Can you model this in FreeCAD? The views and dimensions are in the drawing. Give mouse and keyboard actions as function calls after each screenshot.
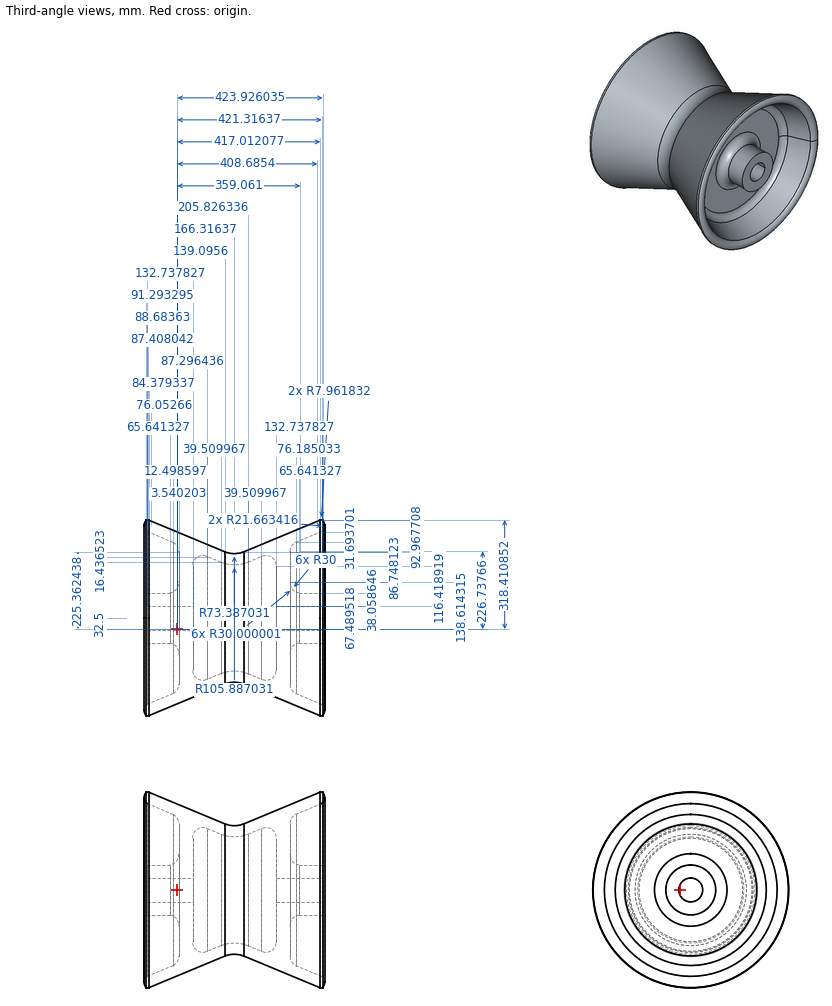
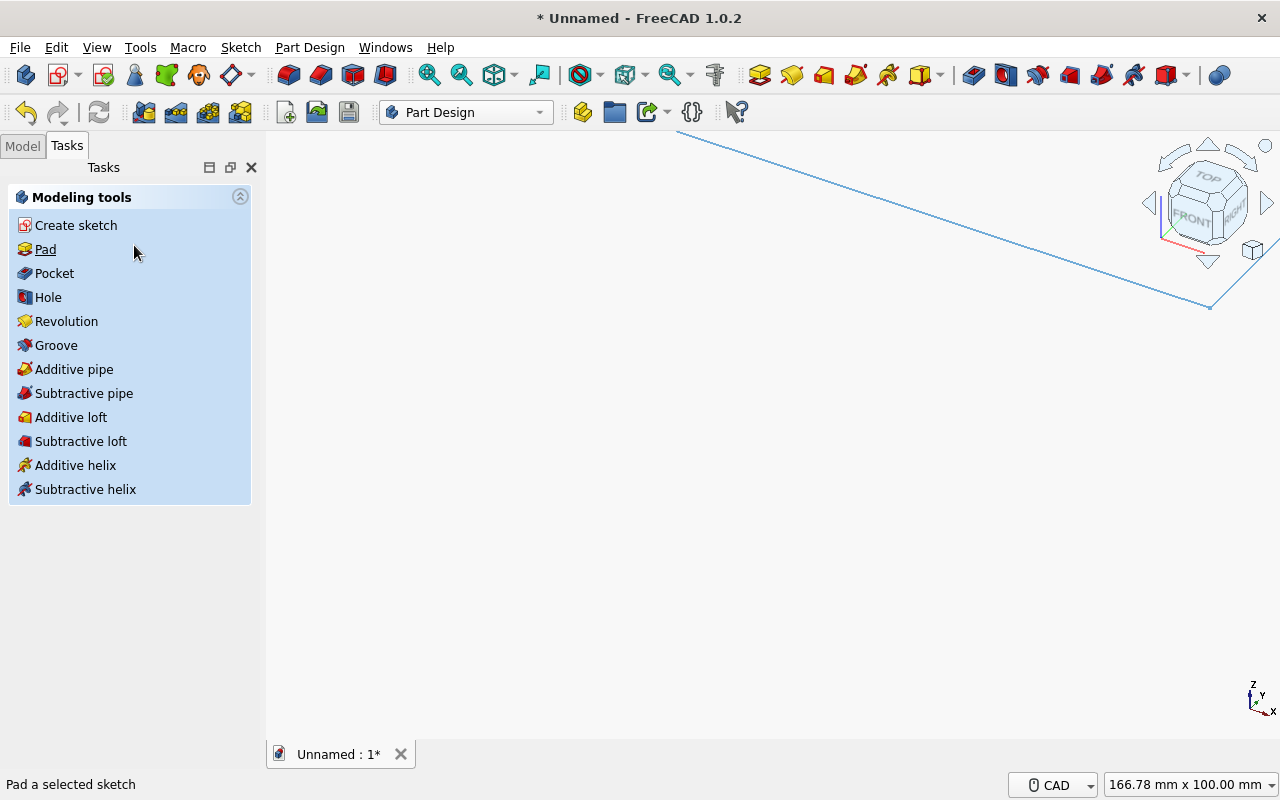
click(792, 76)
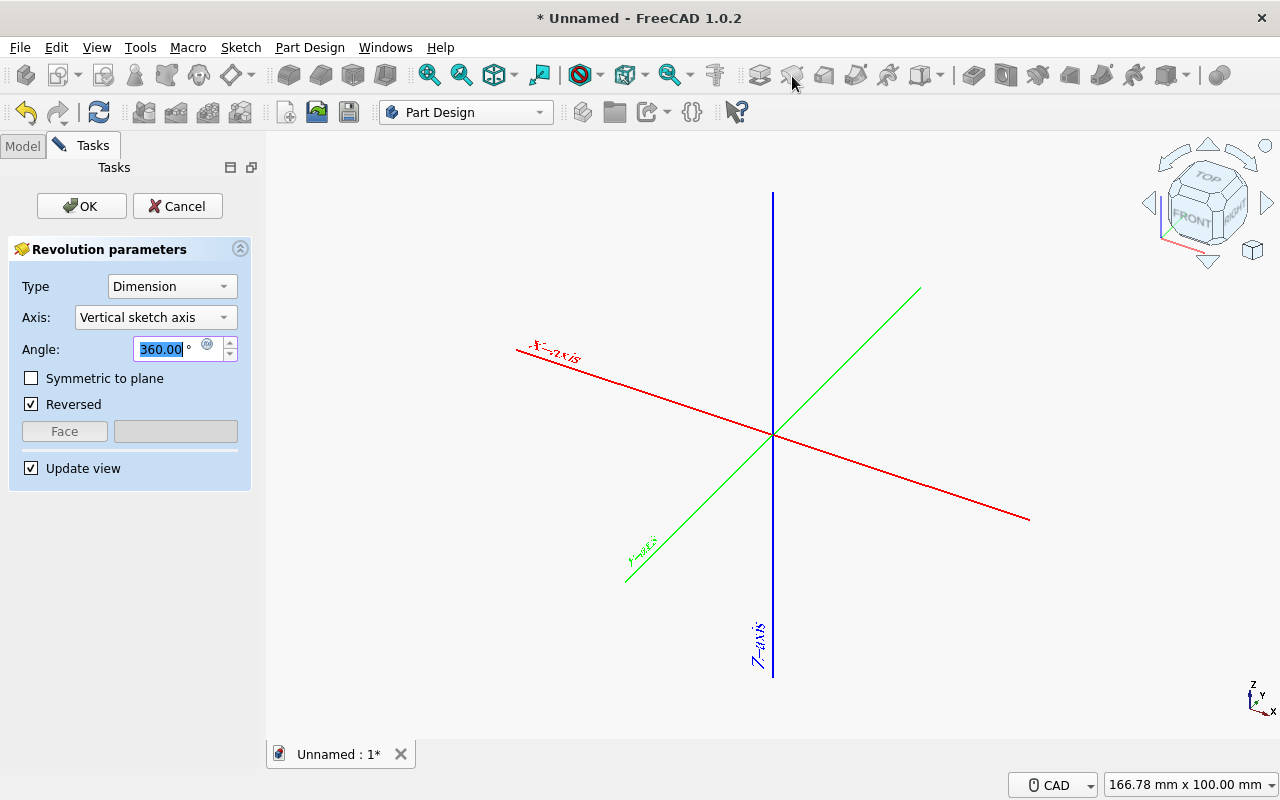
click(156, 318)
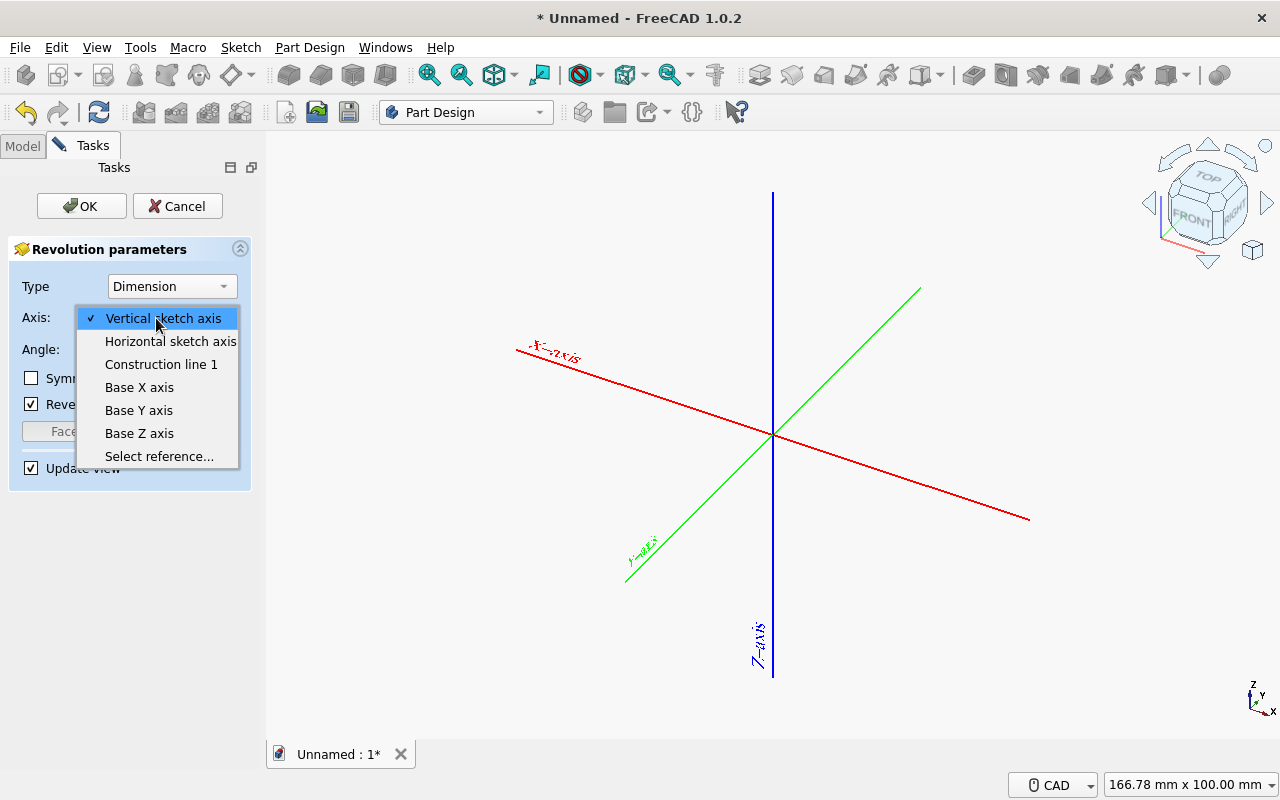
click(156, 364)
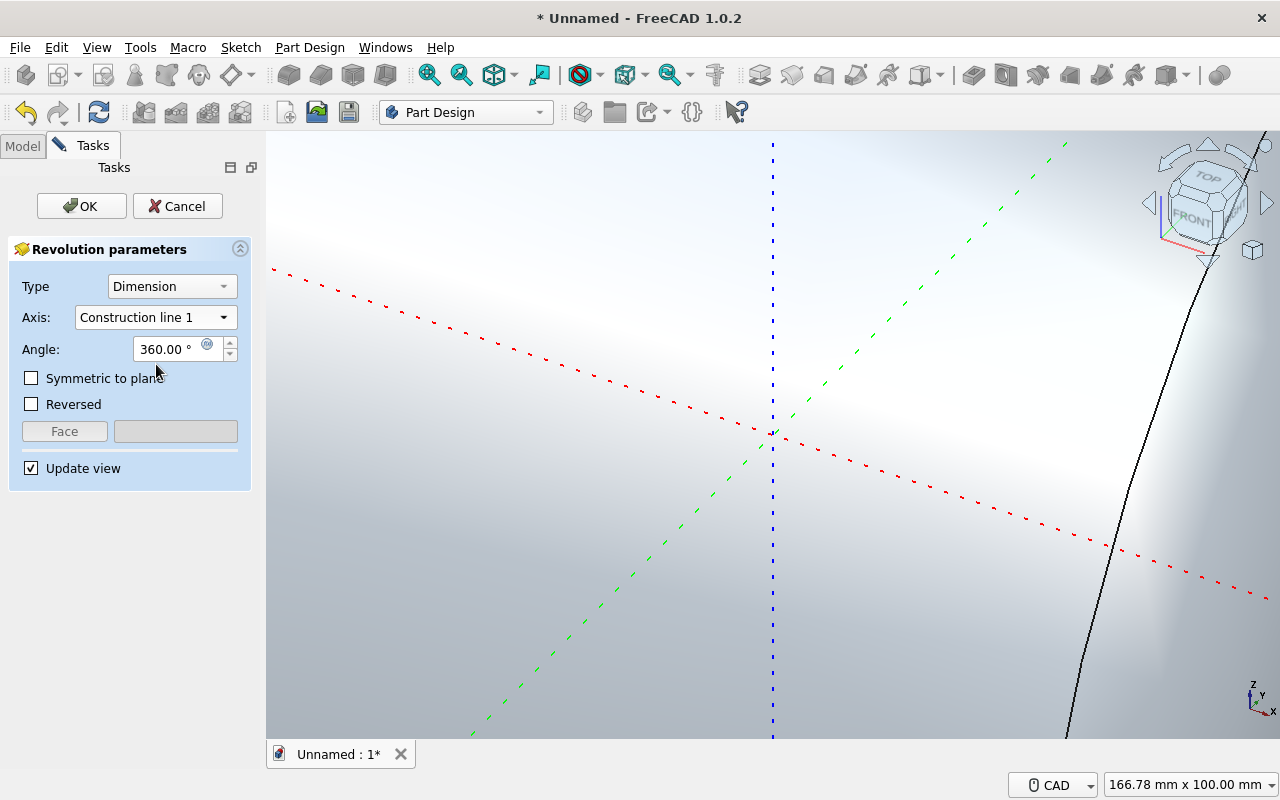
click(82, 206)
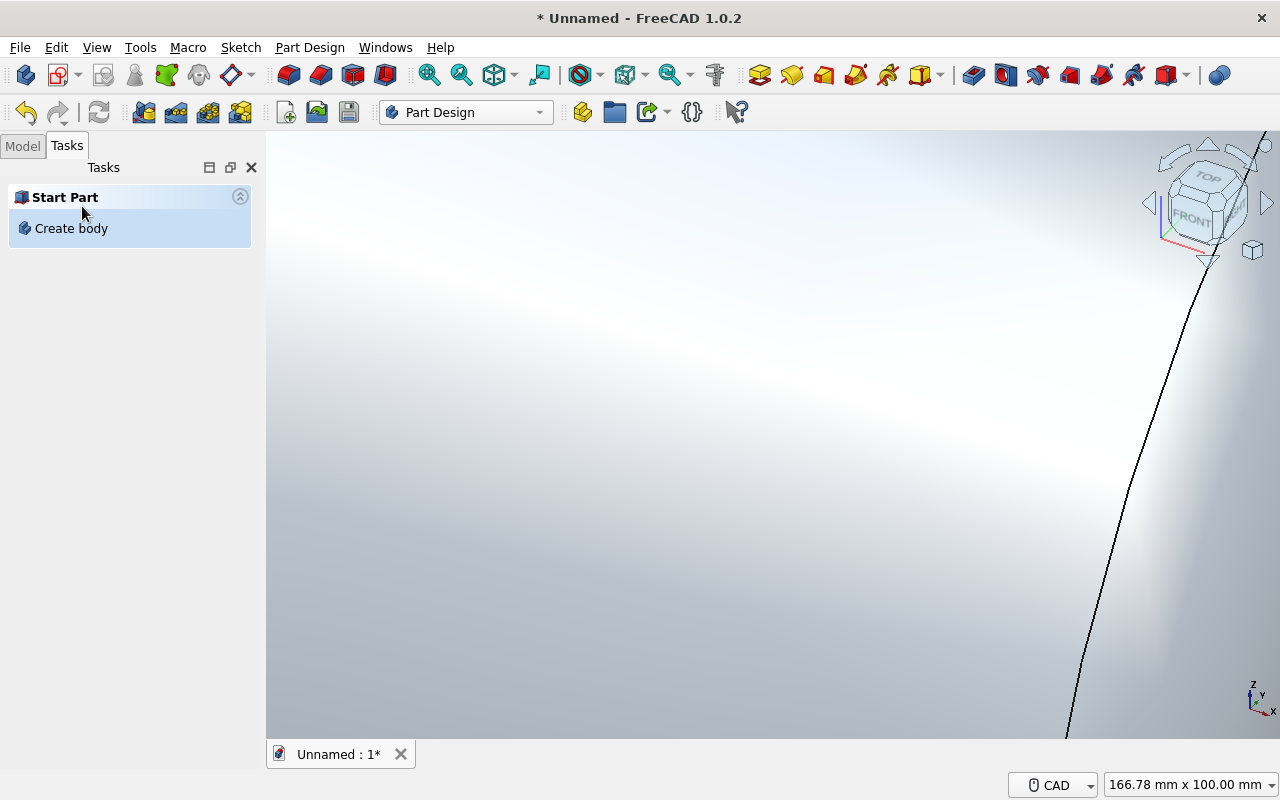
key(0)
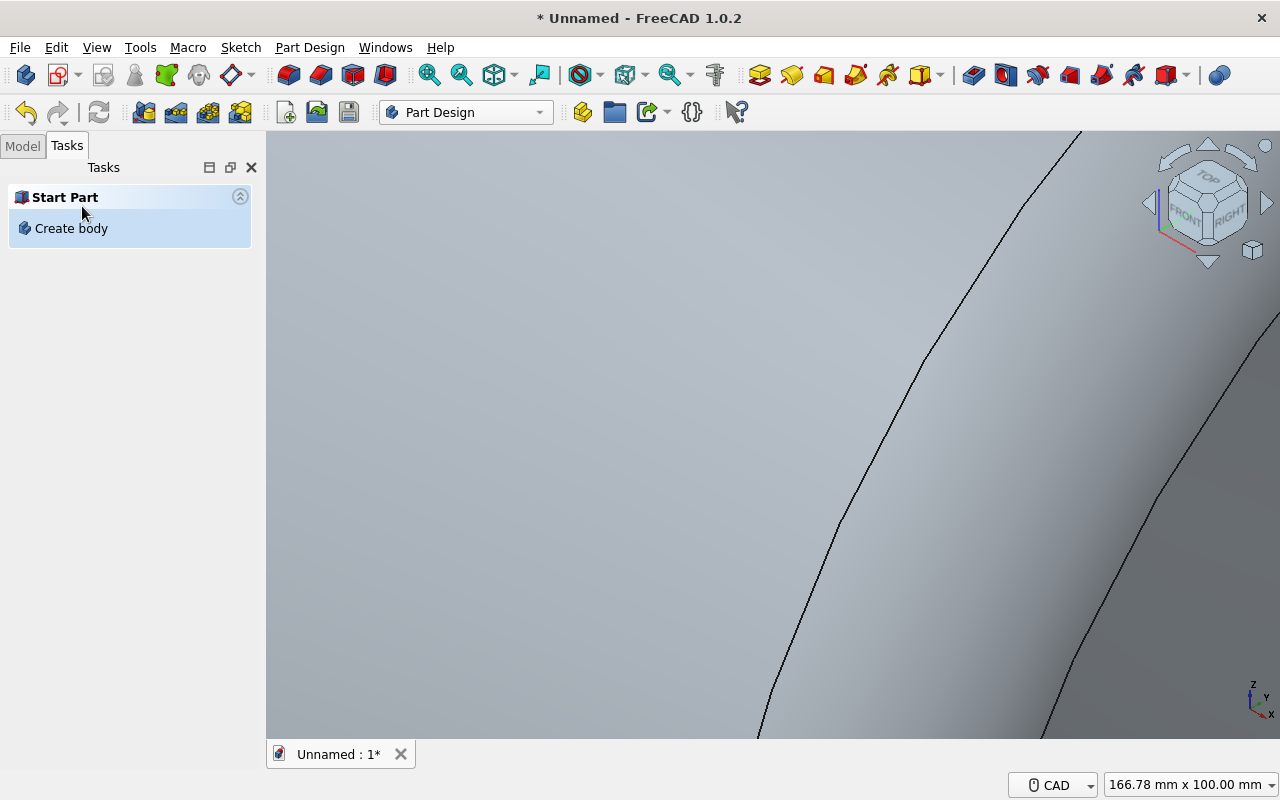
click(430, 76)